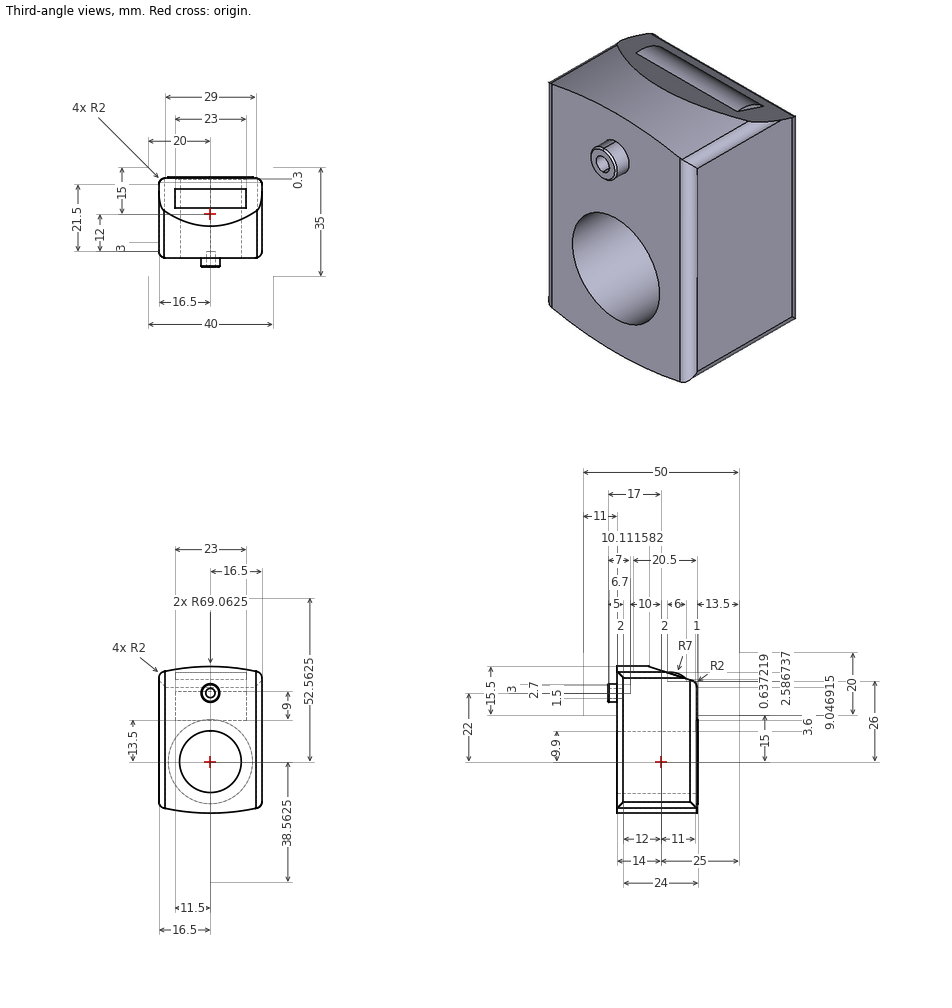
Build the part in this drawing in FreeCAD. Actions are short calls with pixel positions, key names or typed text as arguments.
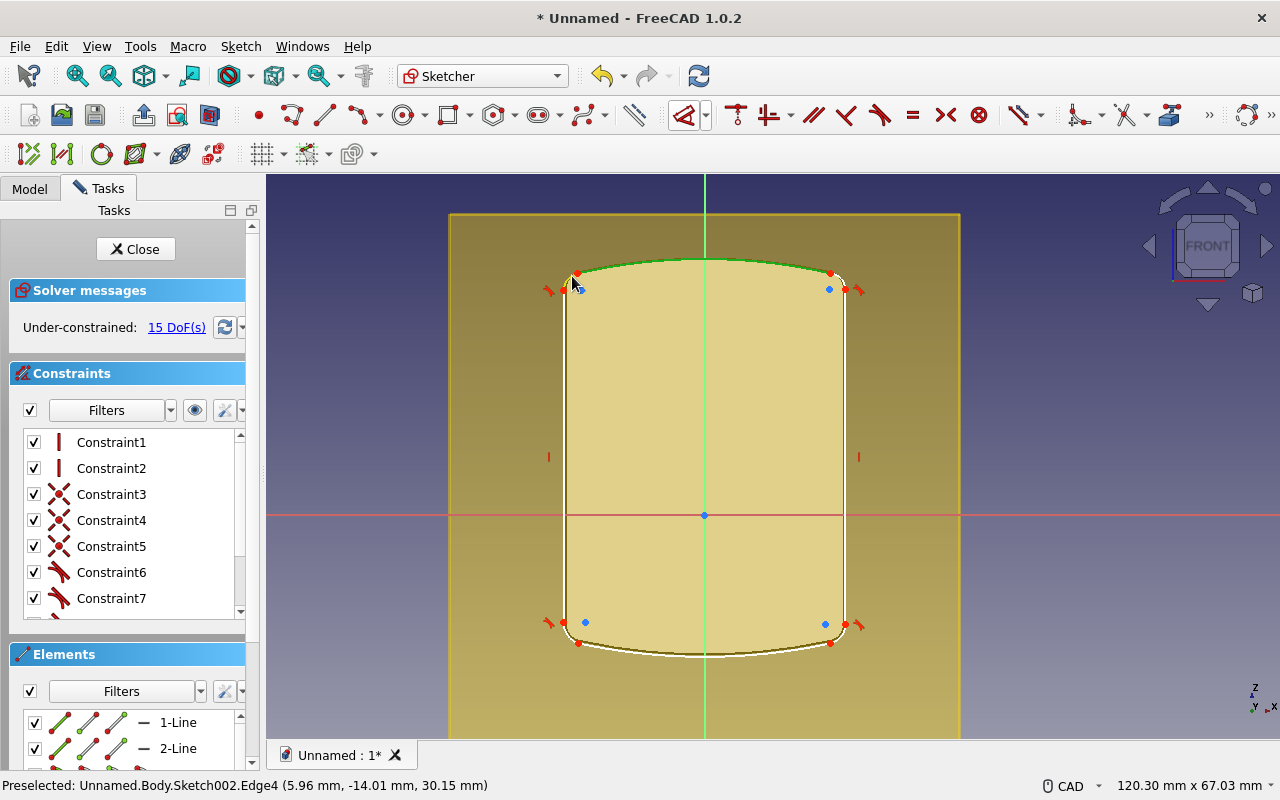
scroll(844, 282, up, 4)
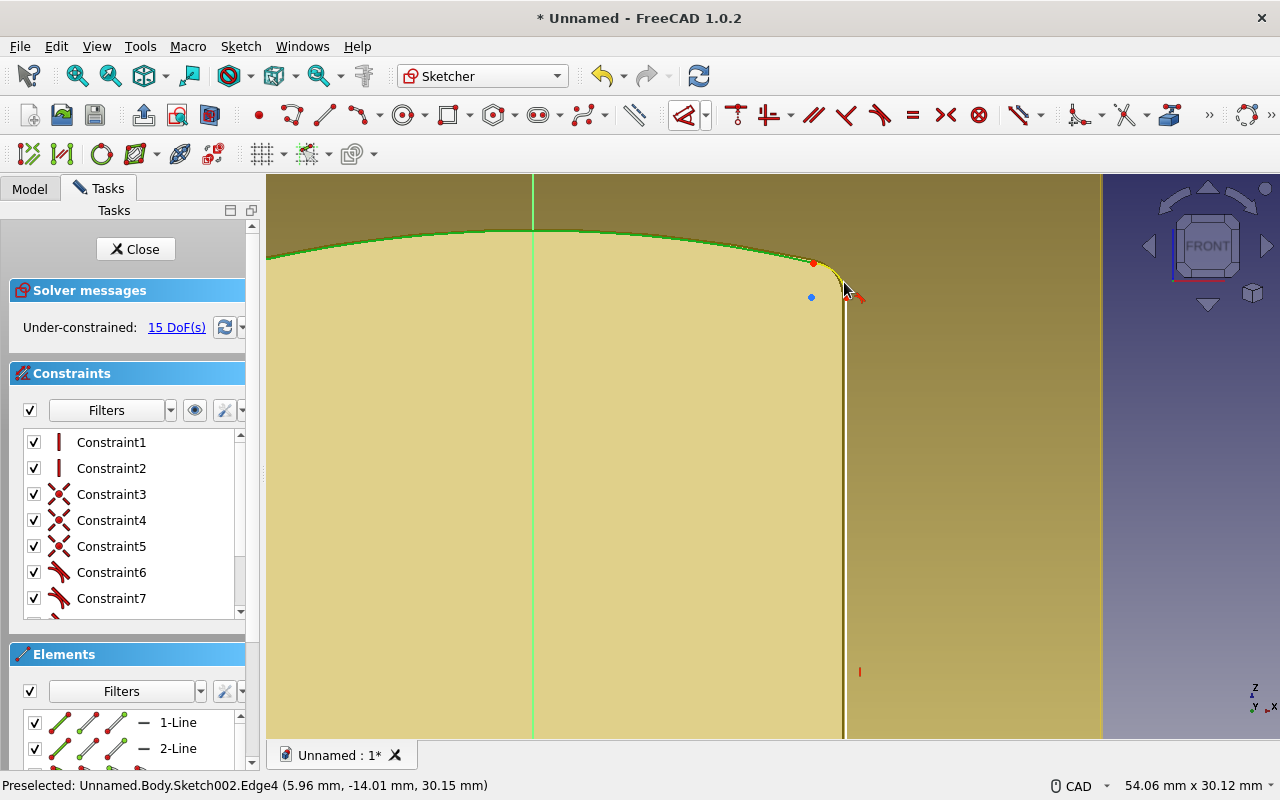
click(843, 283)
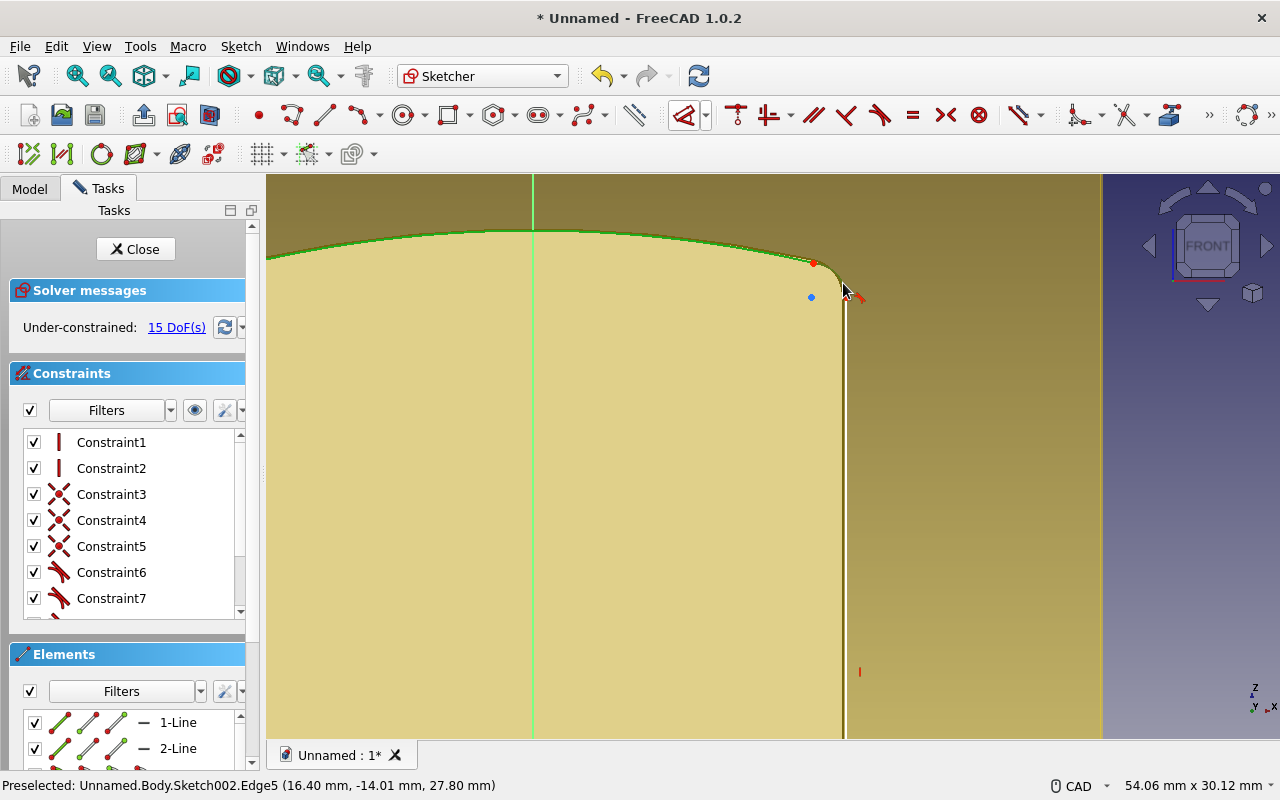
click(880, 116)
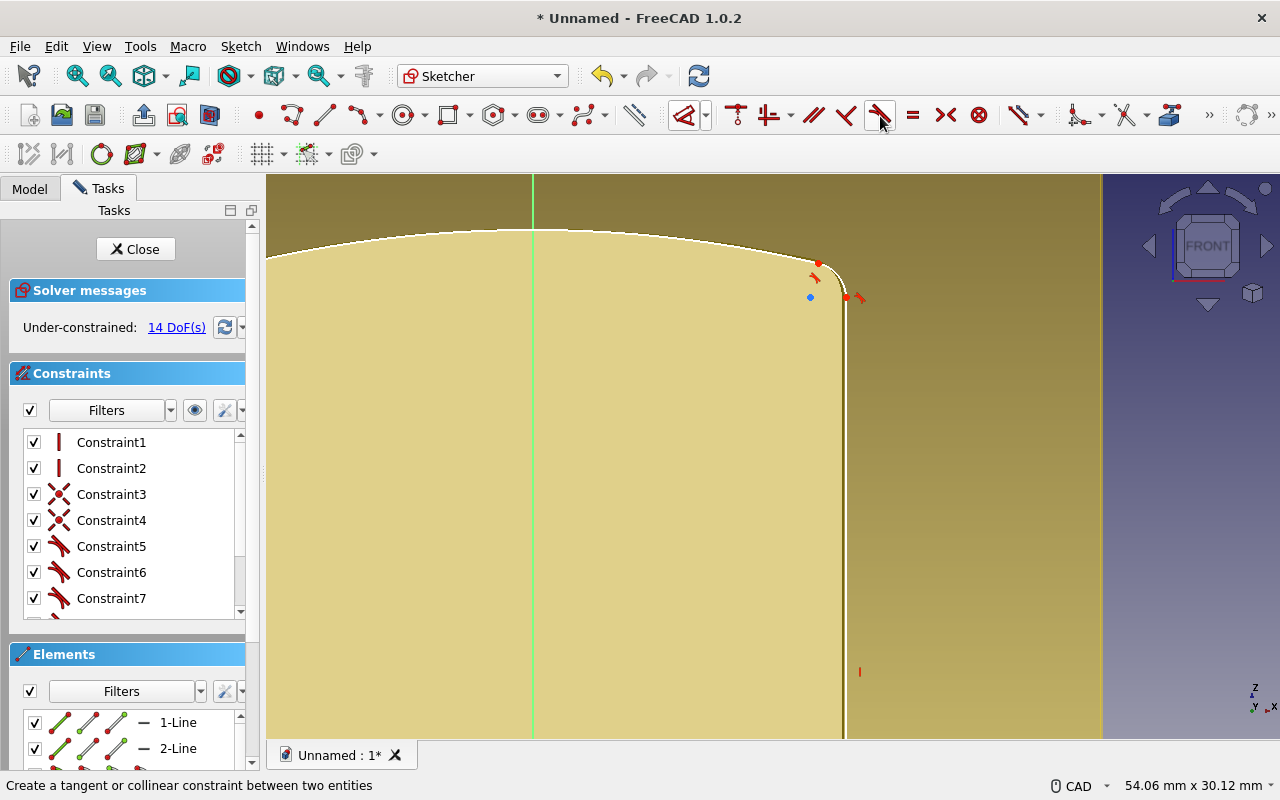
scroll(844, 282, down, 4)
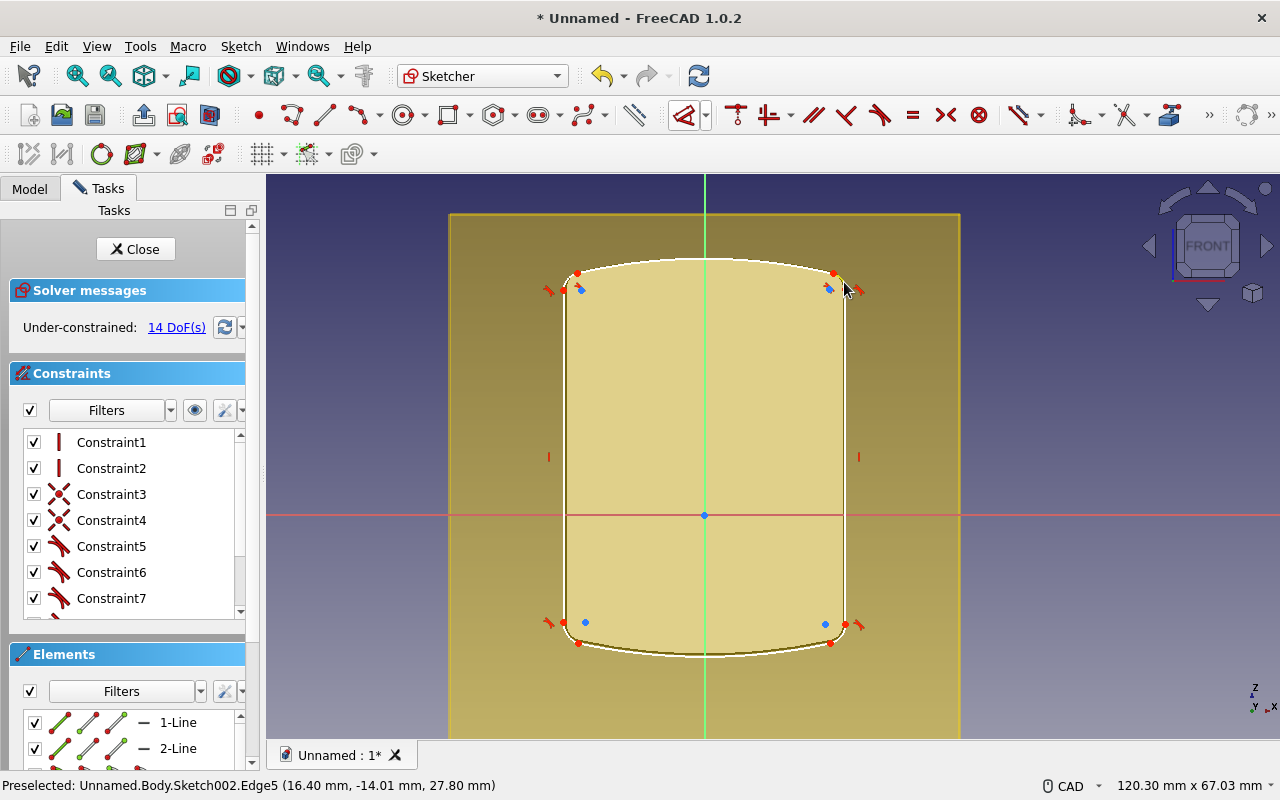
scroll(838, 640, up, 3)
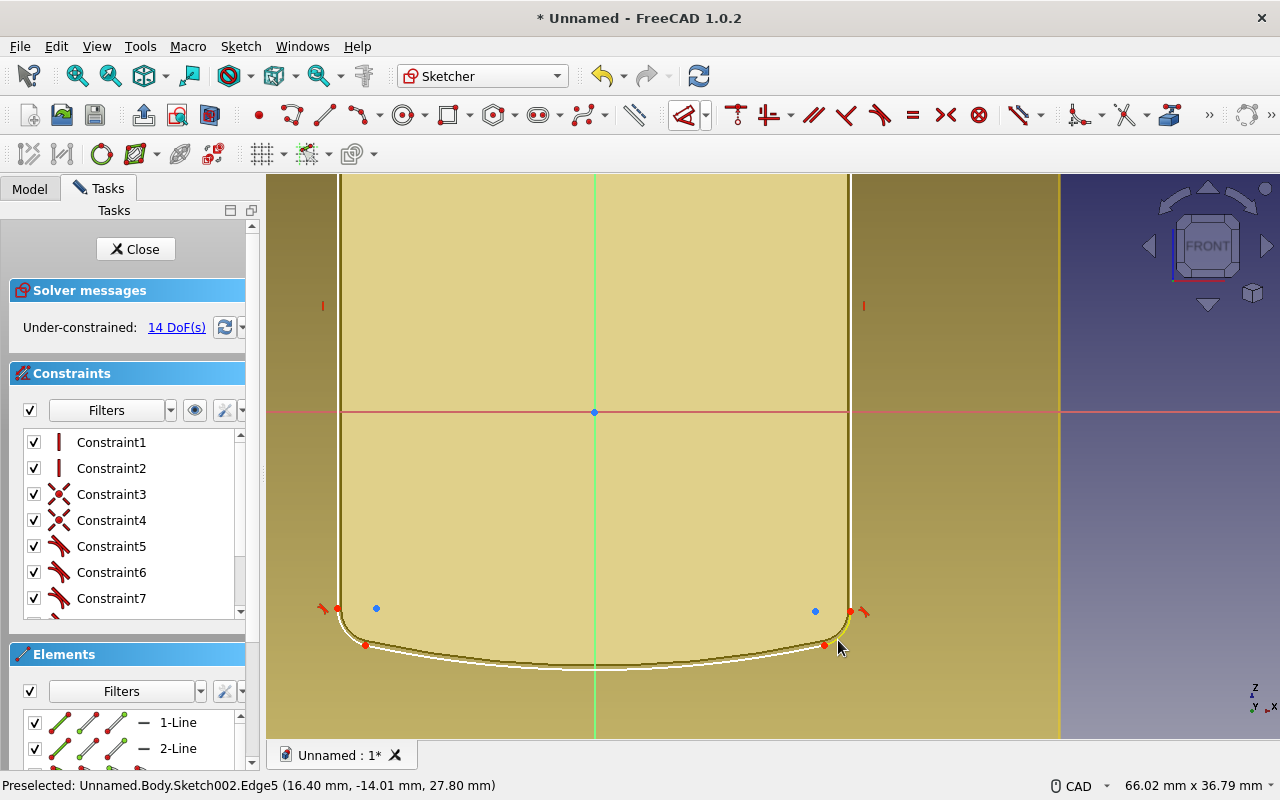
click(837, 639)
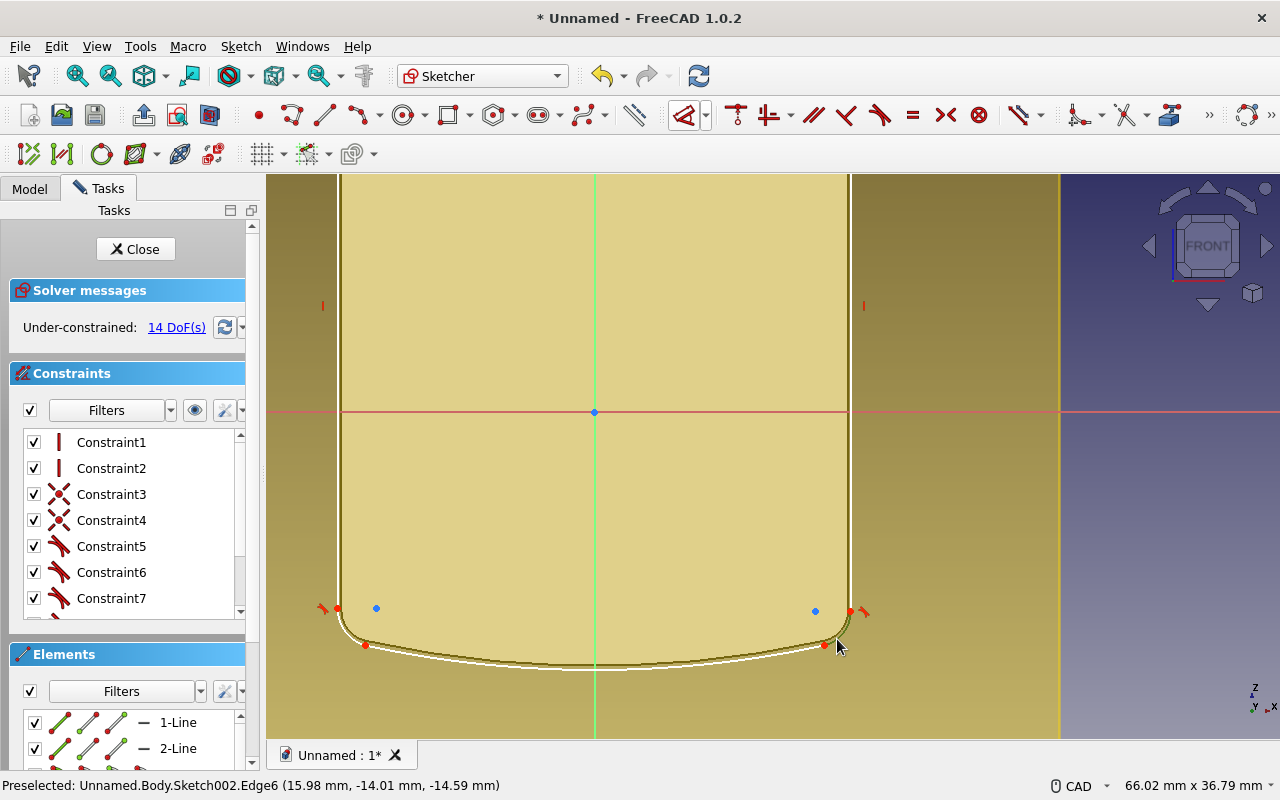
click(502, 666)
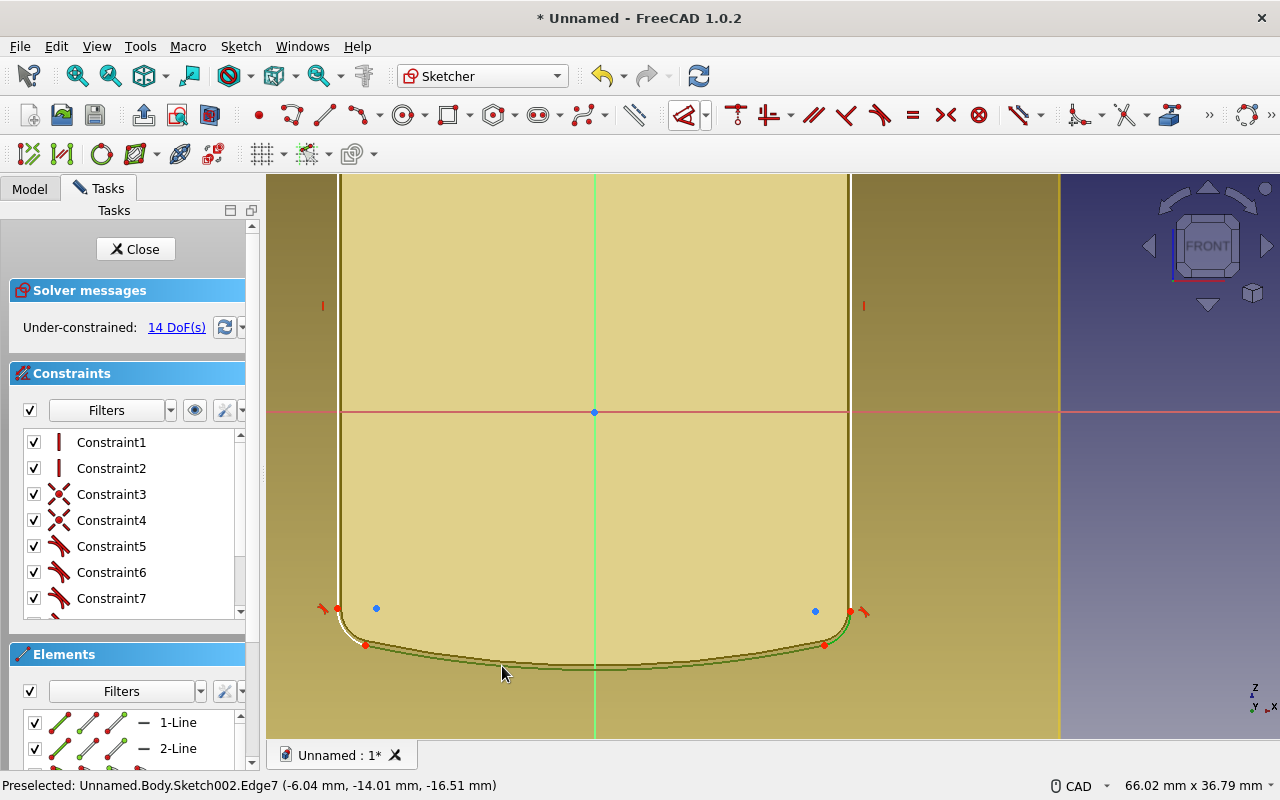
click(880, 116)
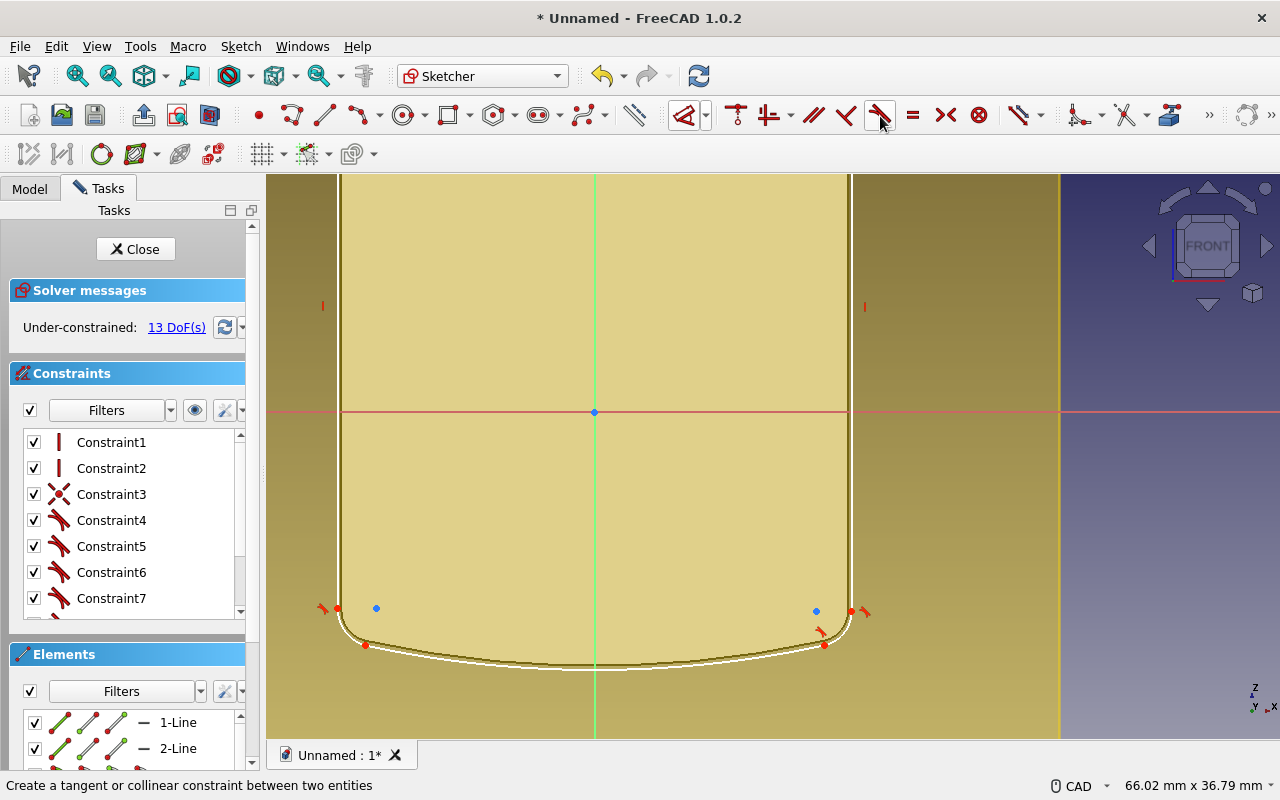
click(502, 666)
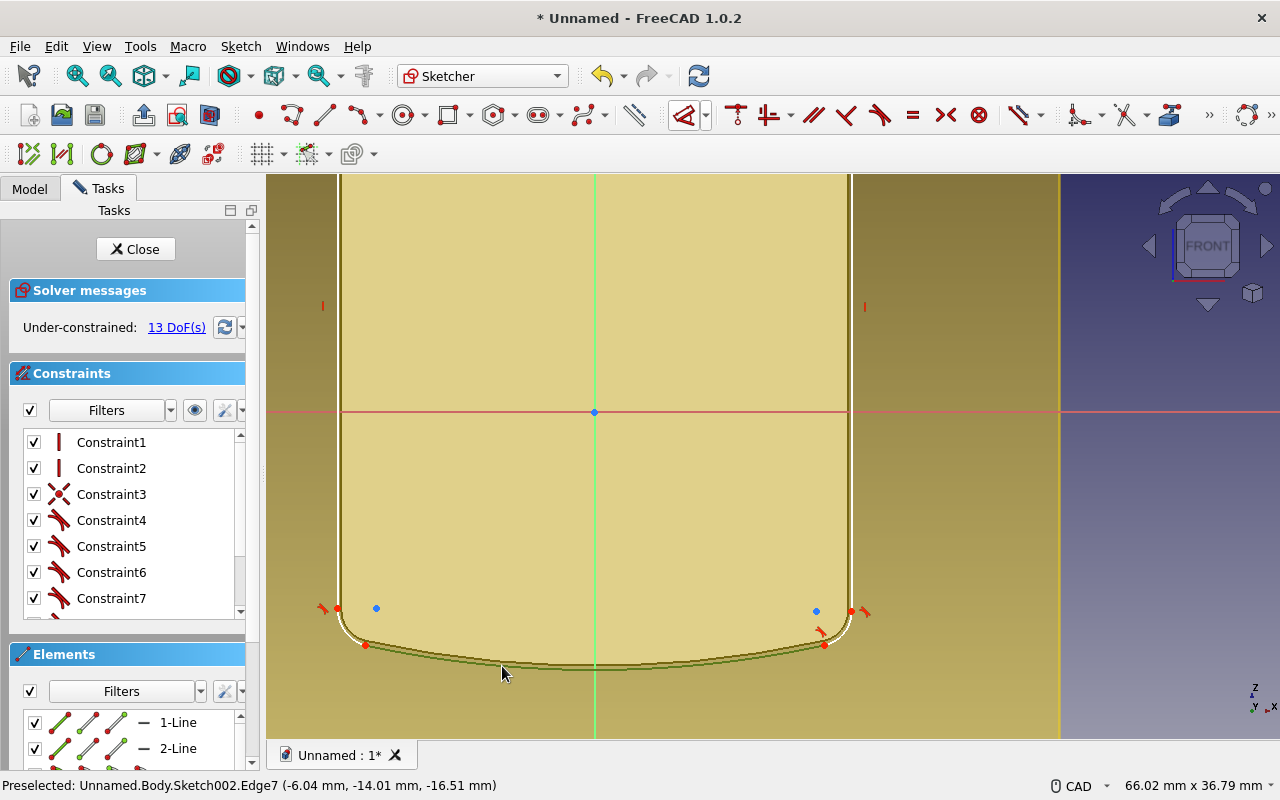
click(341, 623)